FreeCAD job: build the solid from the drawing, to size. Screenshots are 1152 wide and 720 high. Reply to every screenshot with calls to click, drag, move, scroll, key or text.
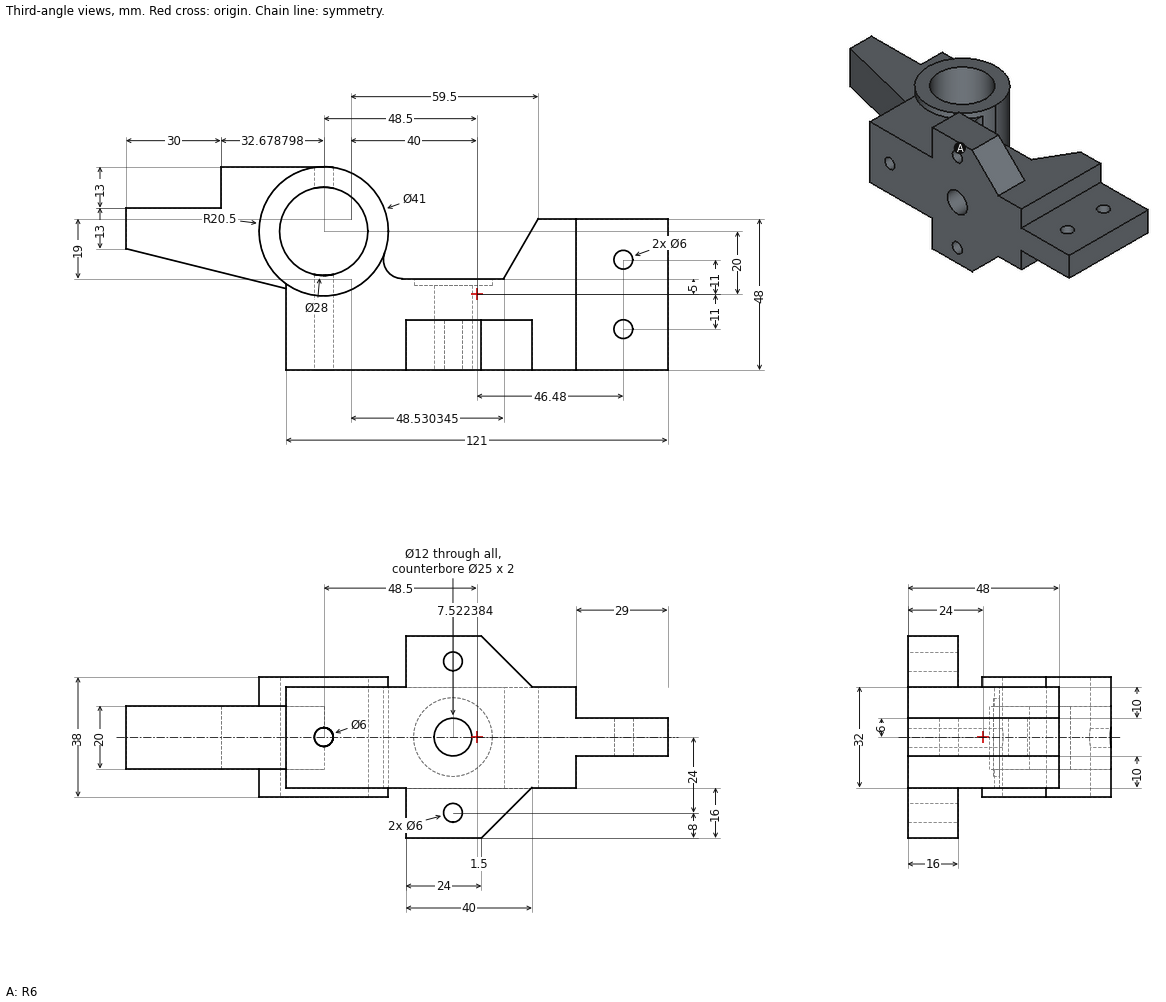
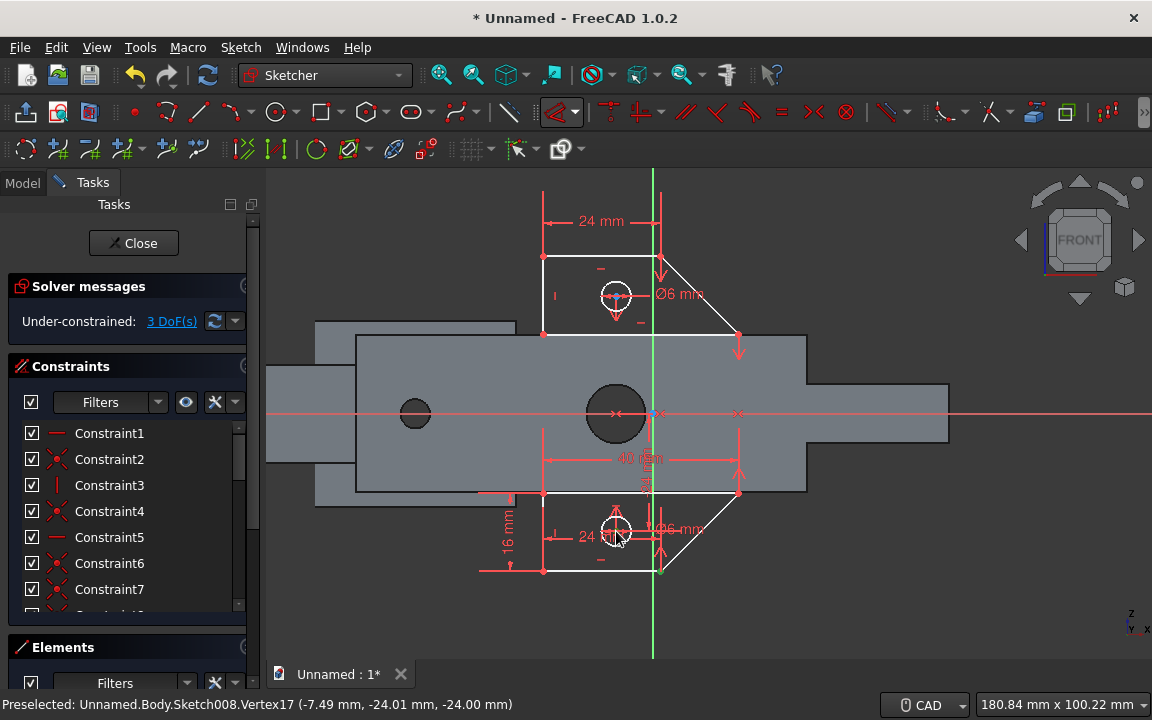
key(i)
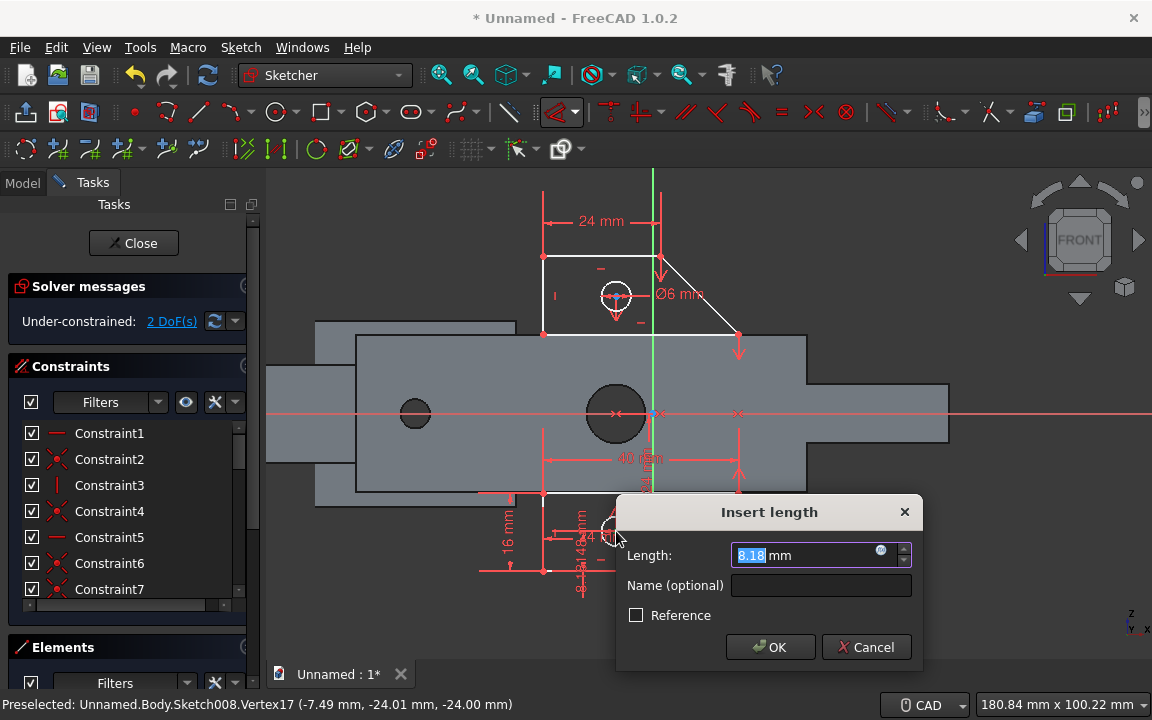
text(8)
key(Return)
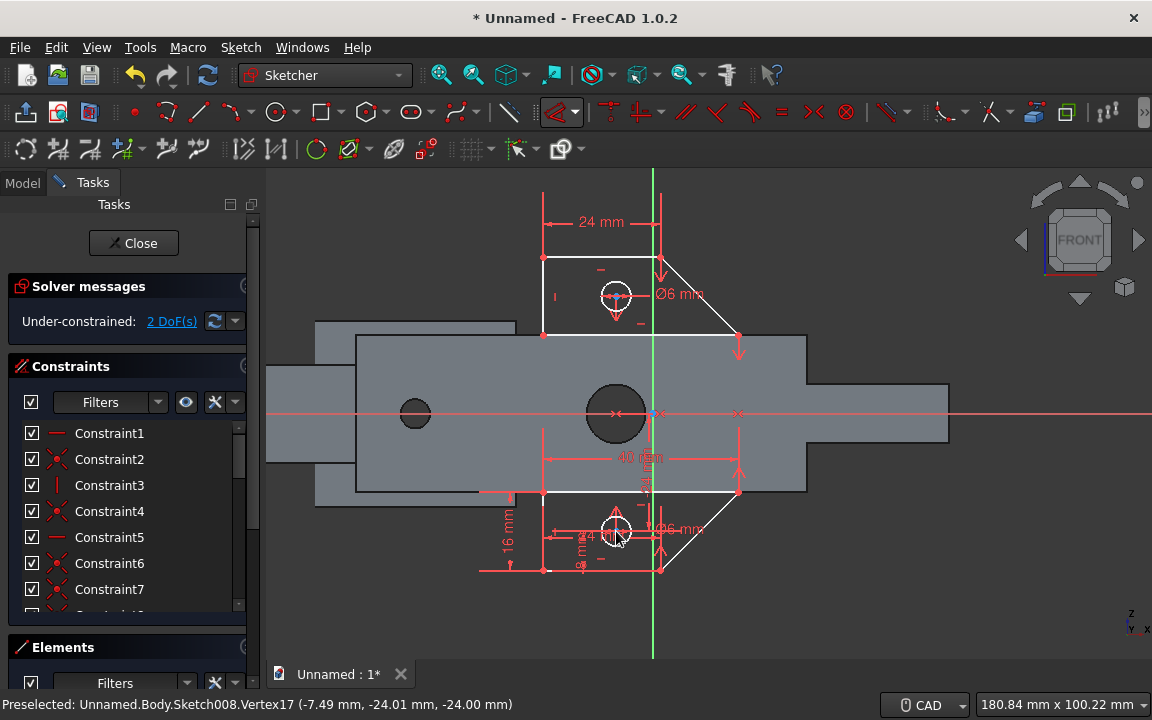
scroll(661, 571, up, 9)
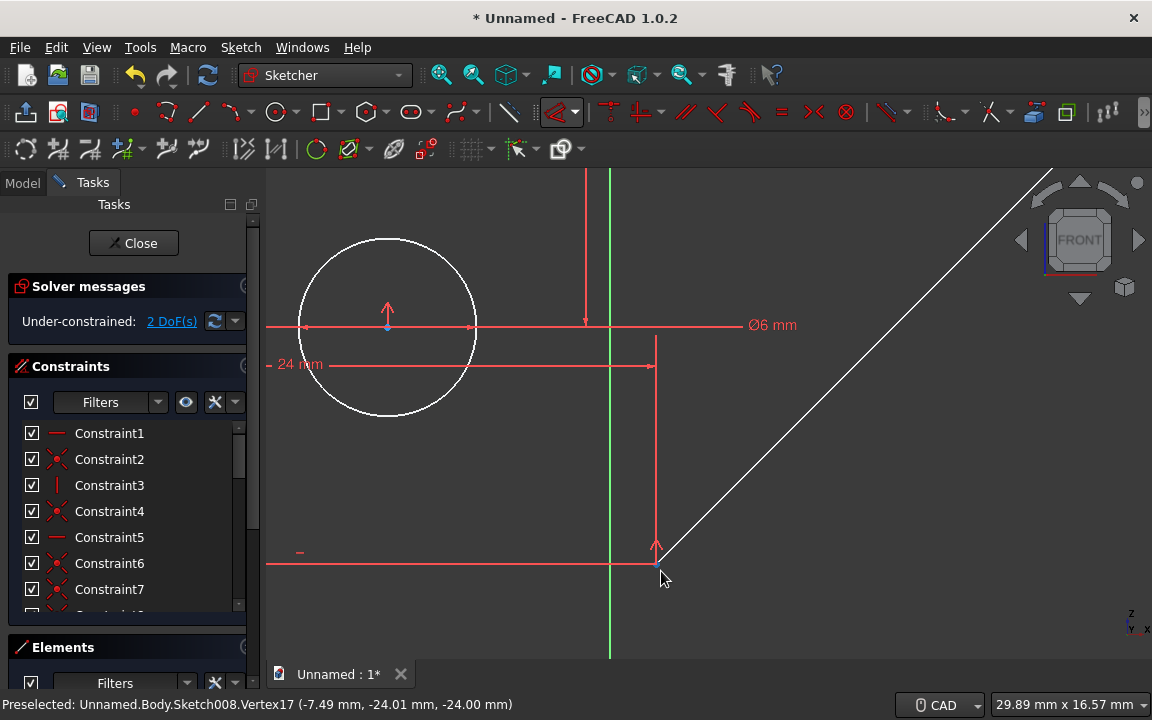
click(656, 564)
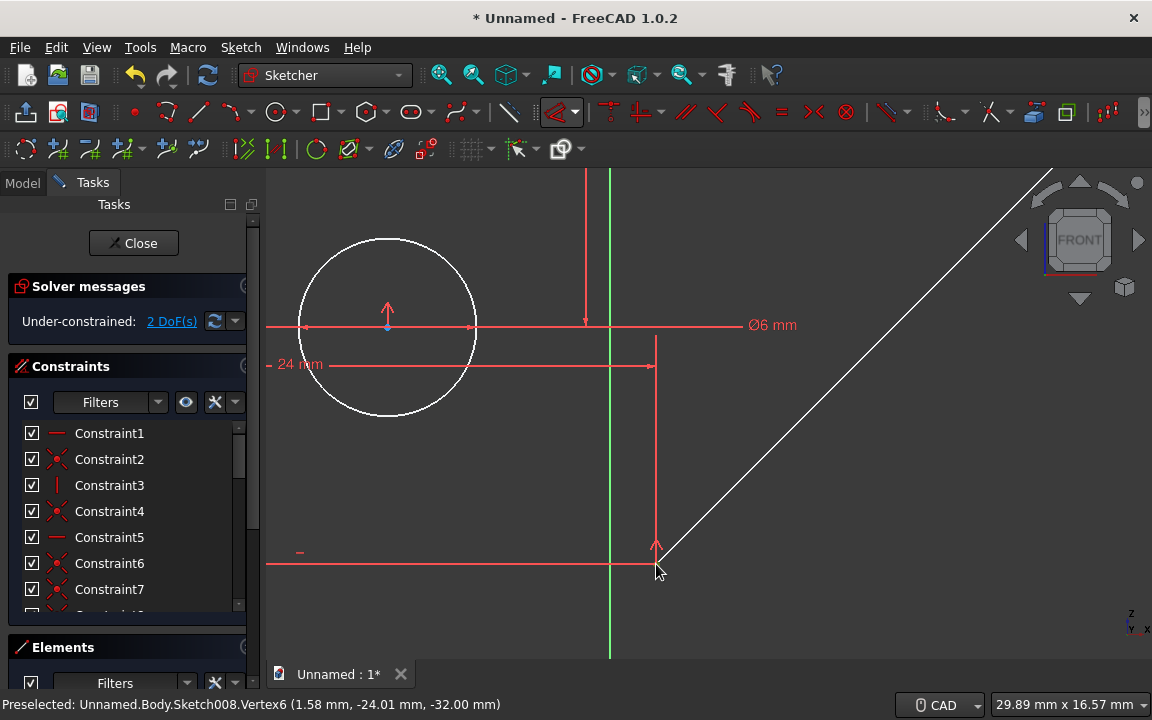
key(l)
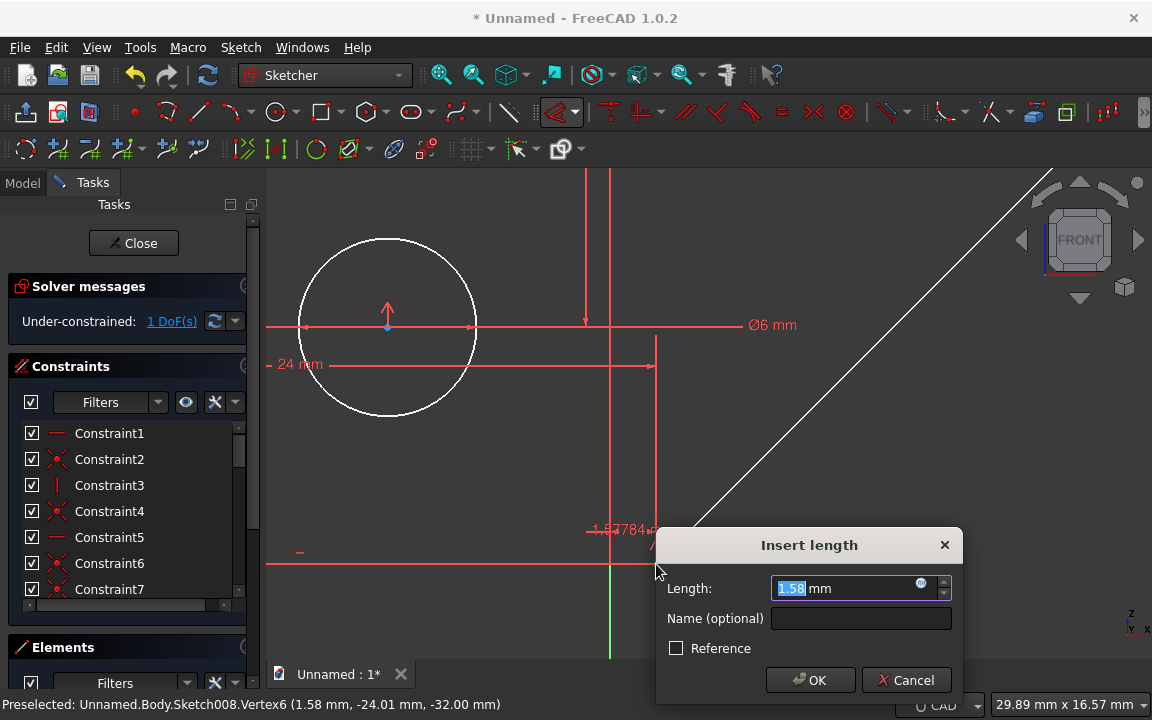
text(1.5)
key(Return)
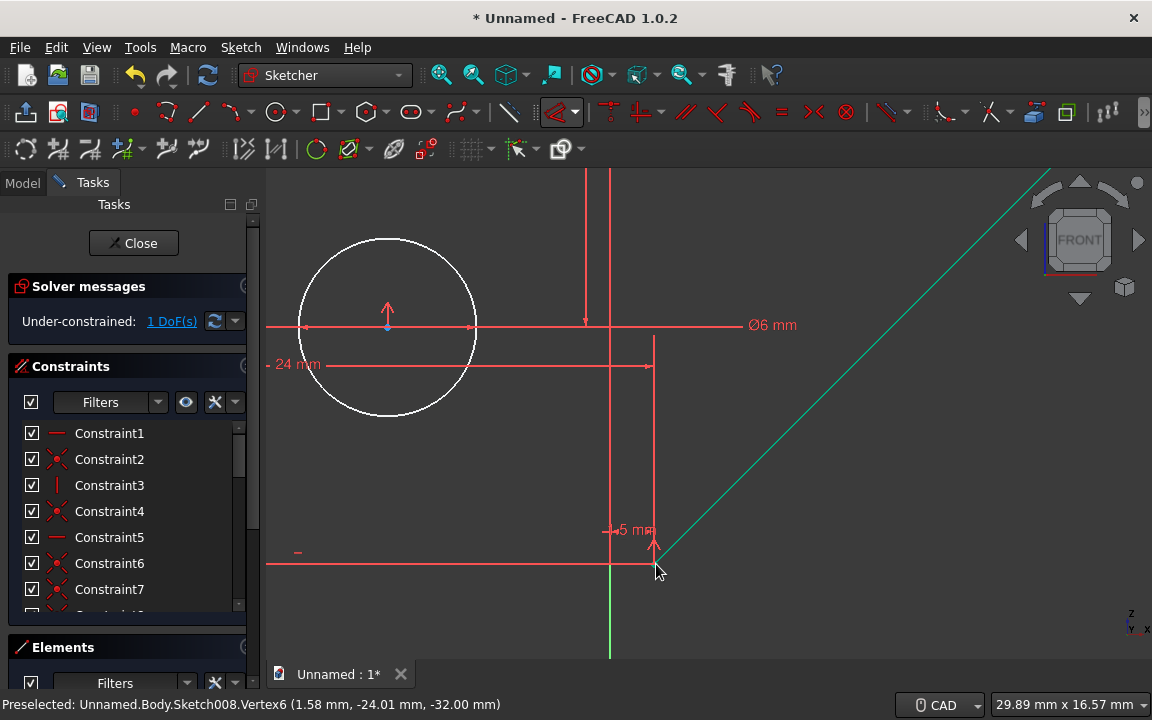
scroll(661, 571, down, 9)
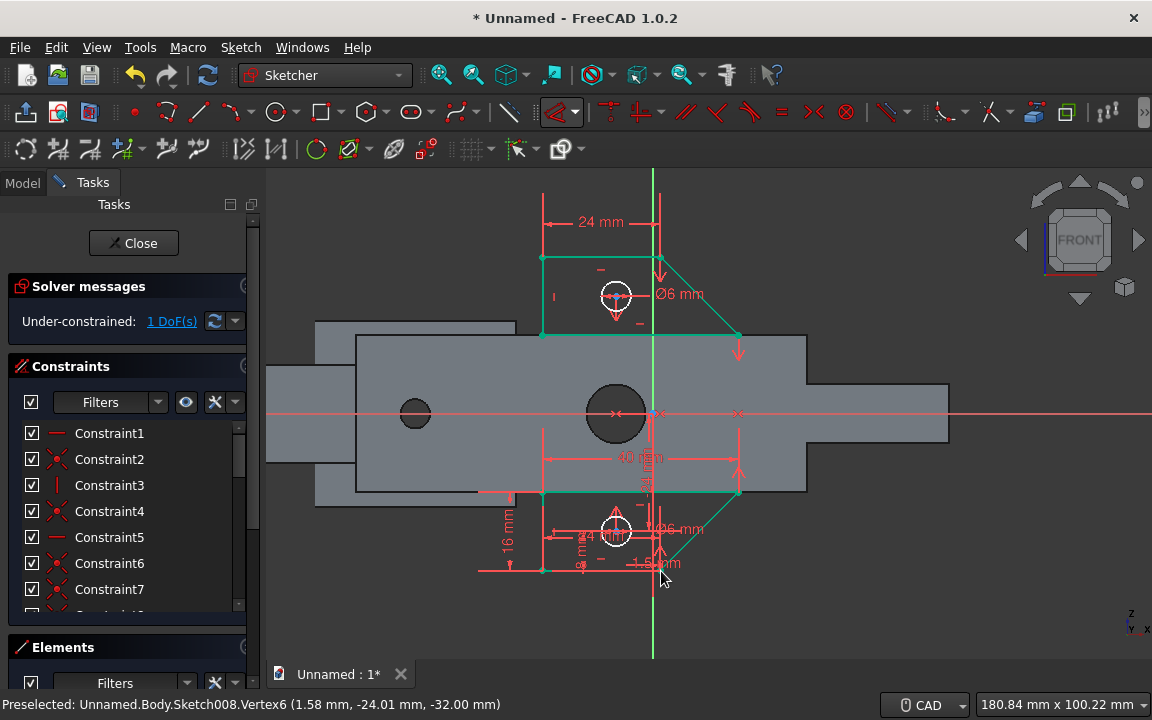
click(616, 531)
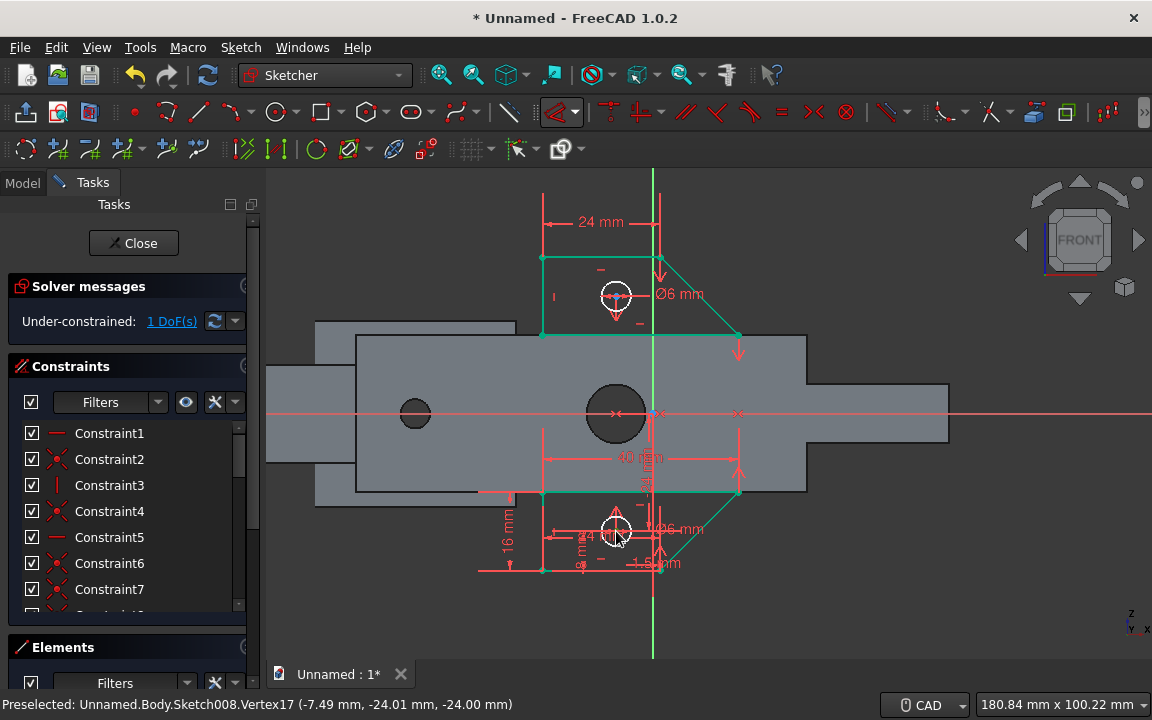
key(l)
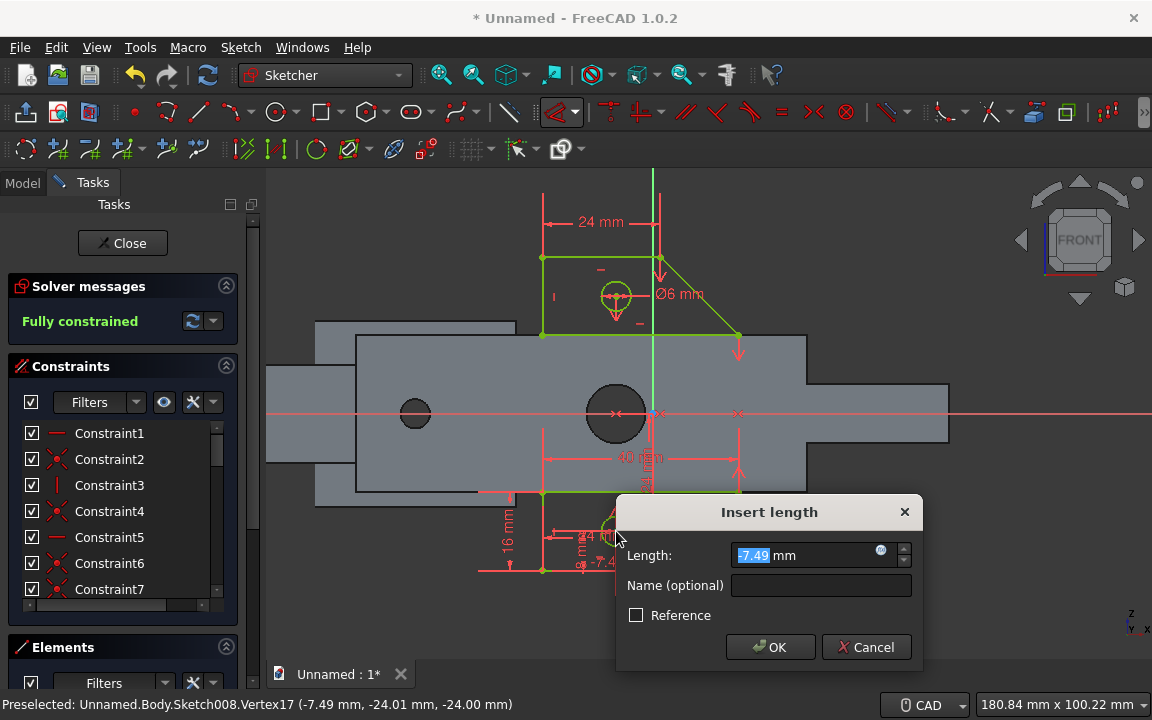
text(-7.522384)
key(Return)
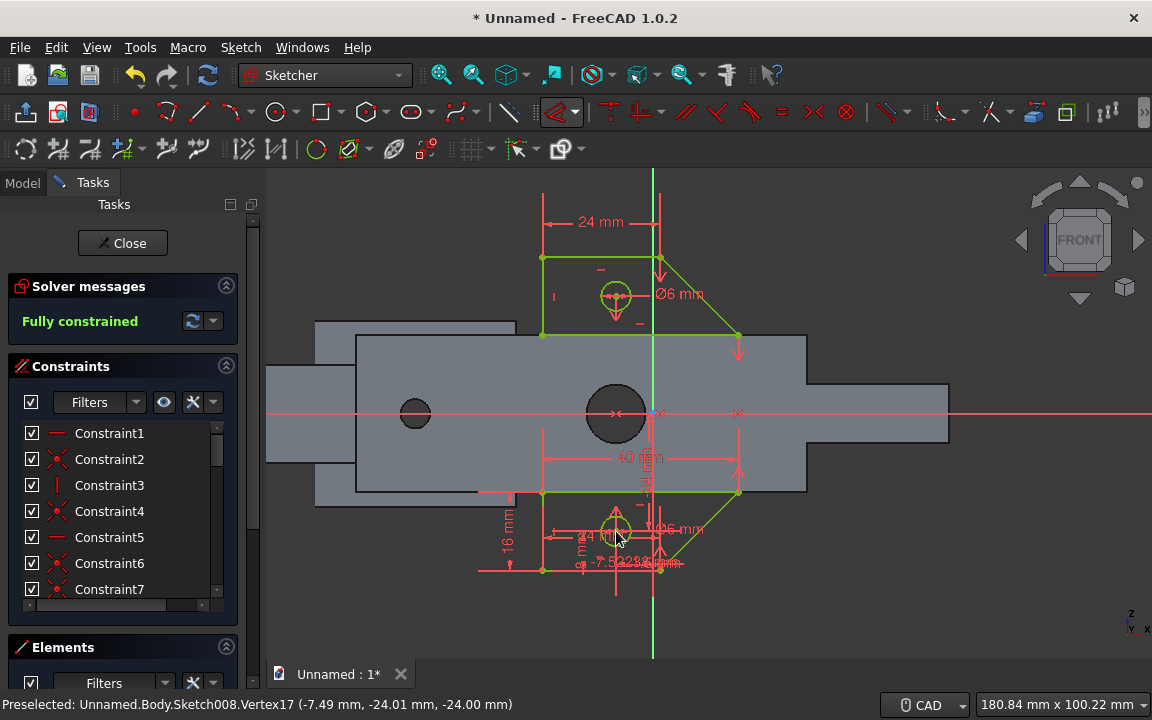
click(123, 243)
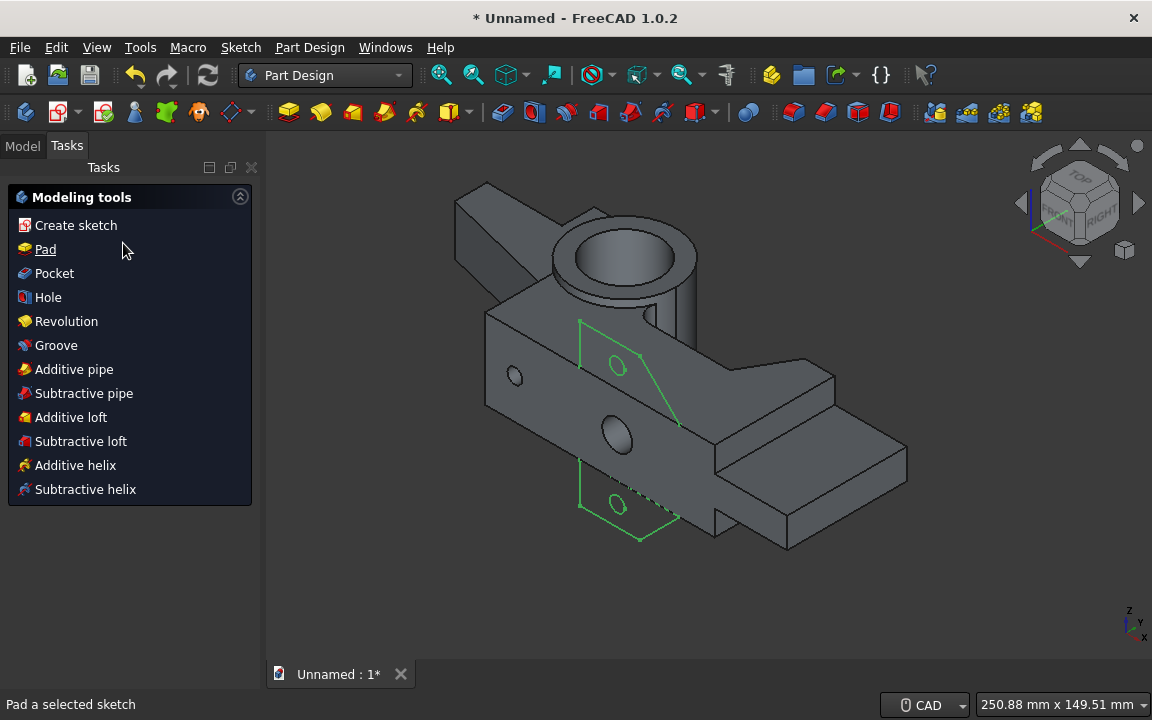
click(290, 112)